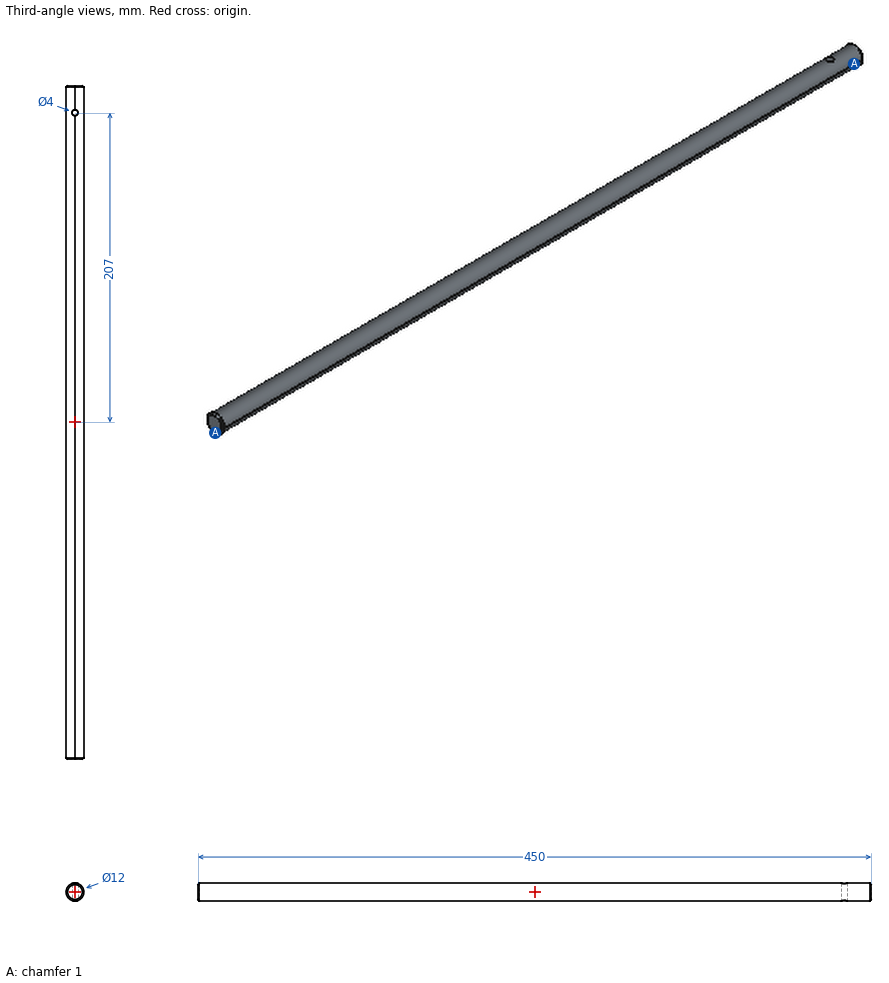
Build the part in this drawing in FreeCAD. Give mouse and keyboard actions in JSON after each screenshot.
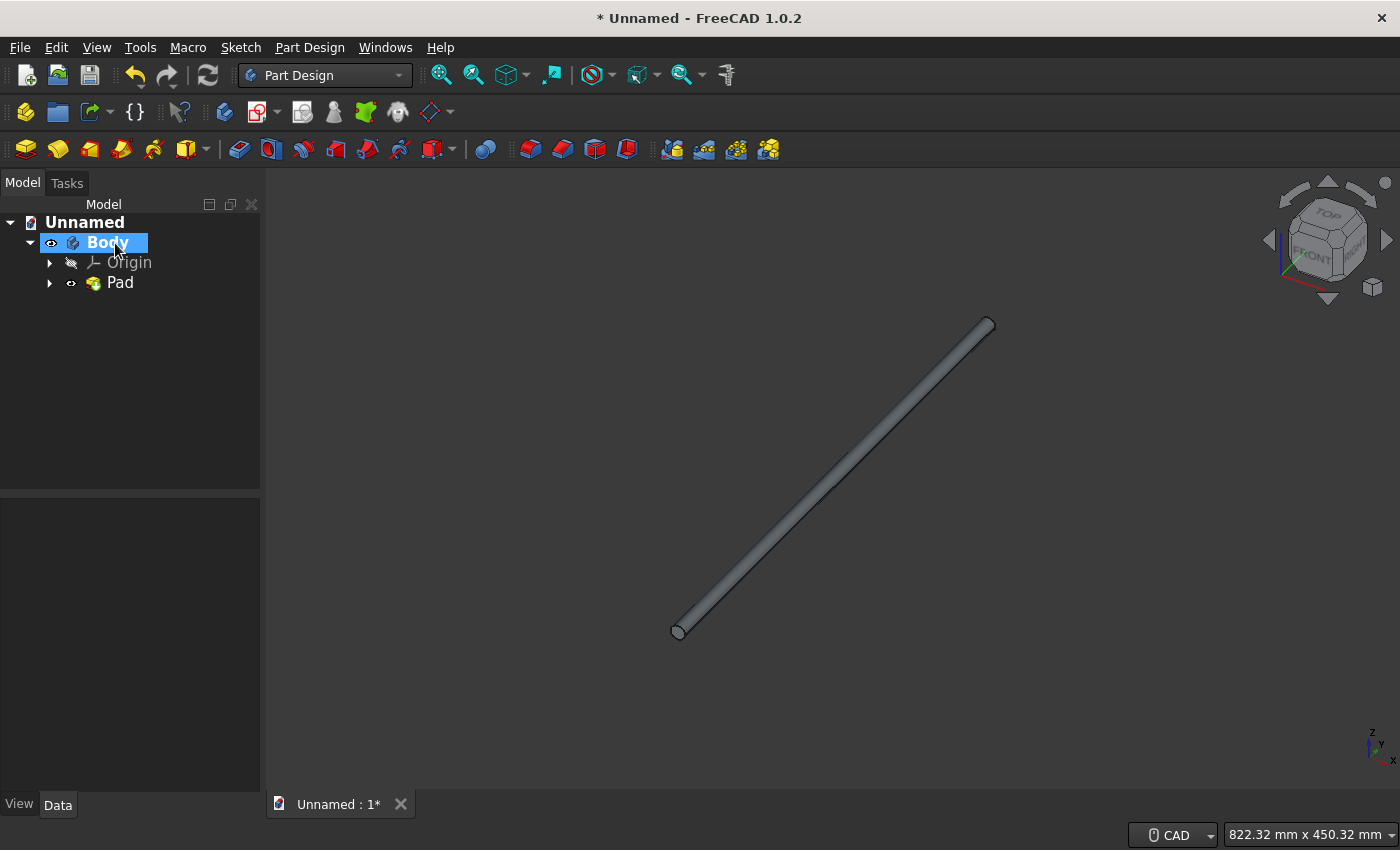
{"action": "left_click", "coordinate": [671, 629]}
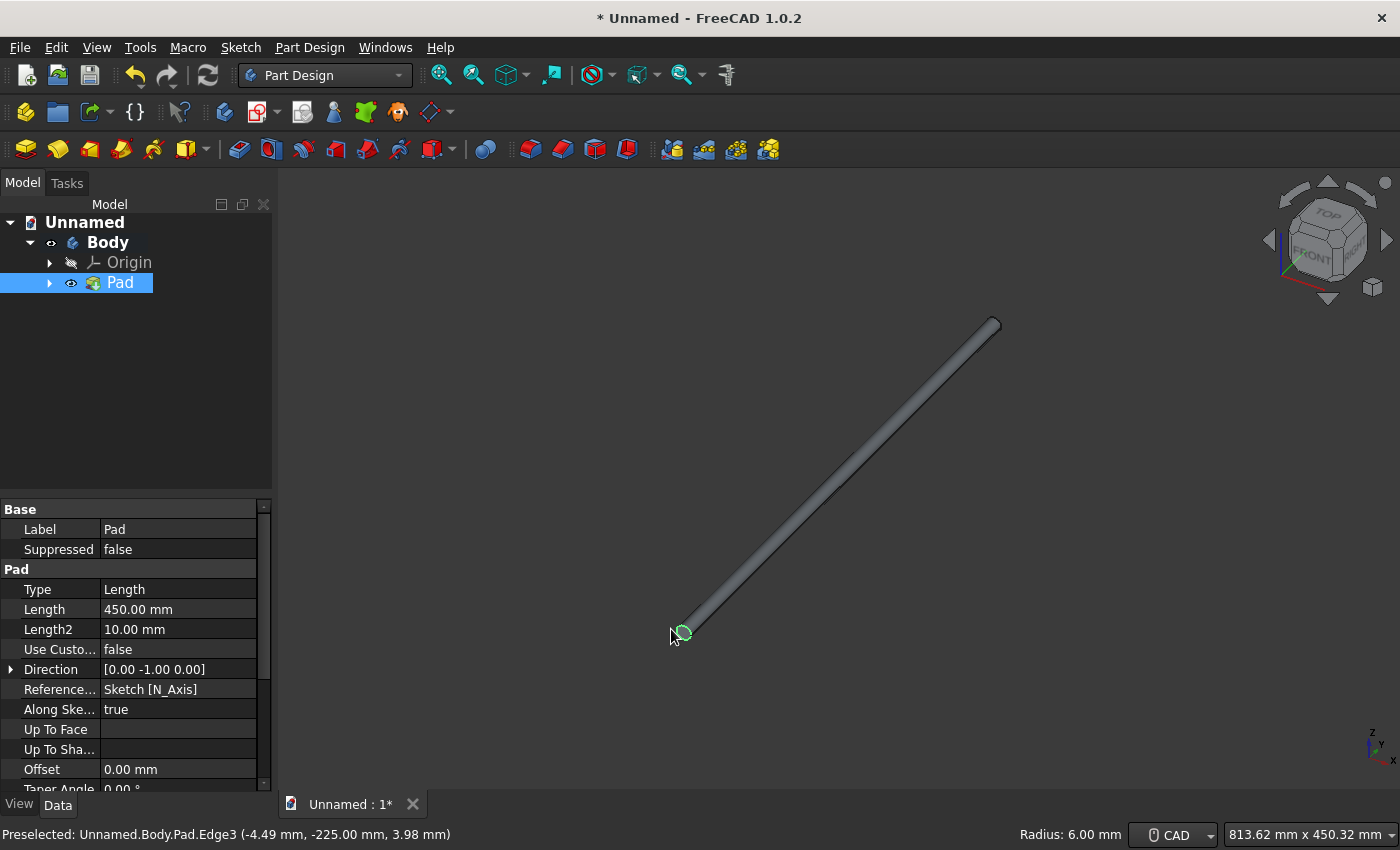
{"action": "left_click", "coordinate": [992, 316], "text": "ctrl"}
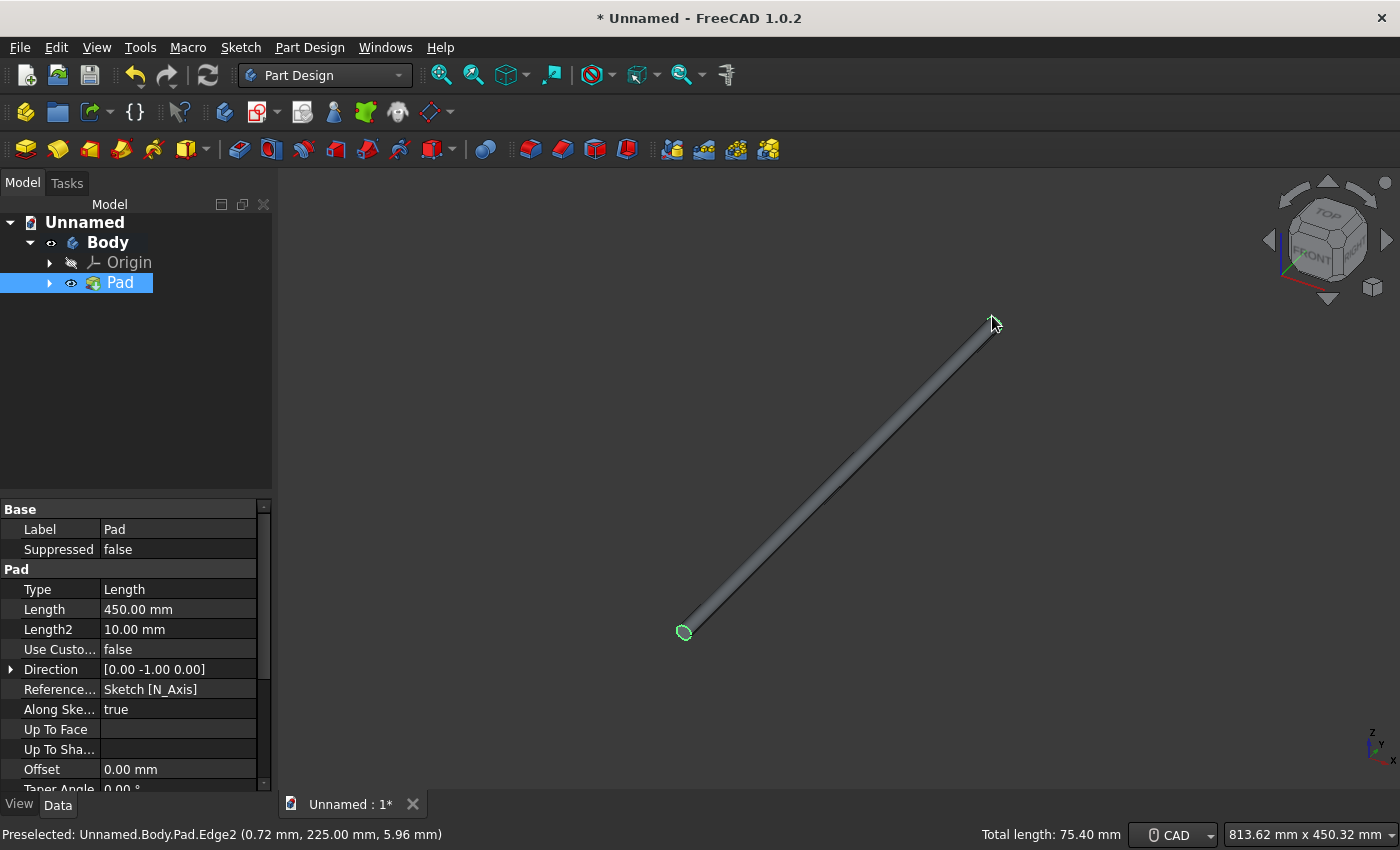
{"action": "left_click", "coordinate": [564, 150]}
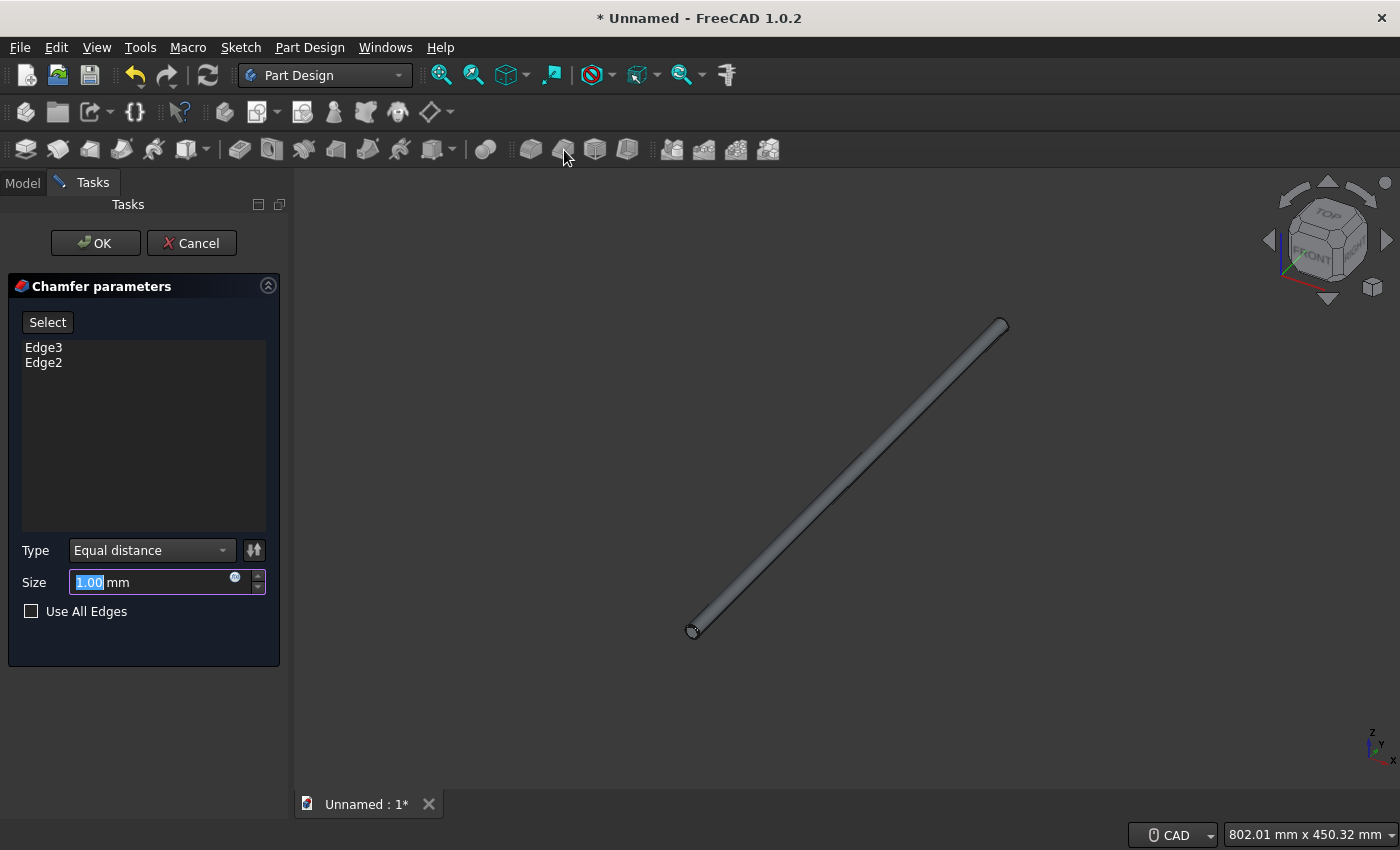
{"action": "type", "text": "1"}
{"action": "key", "text": "Tab"}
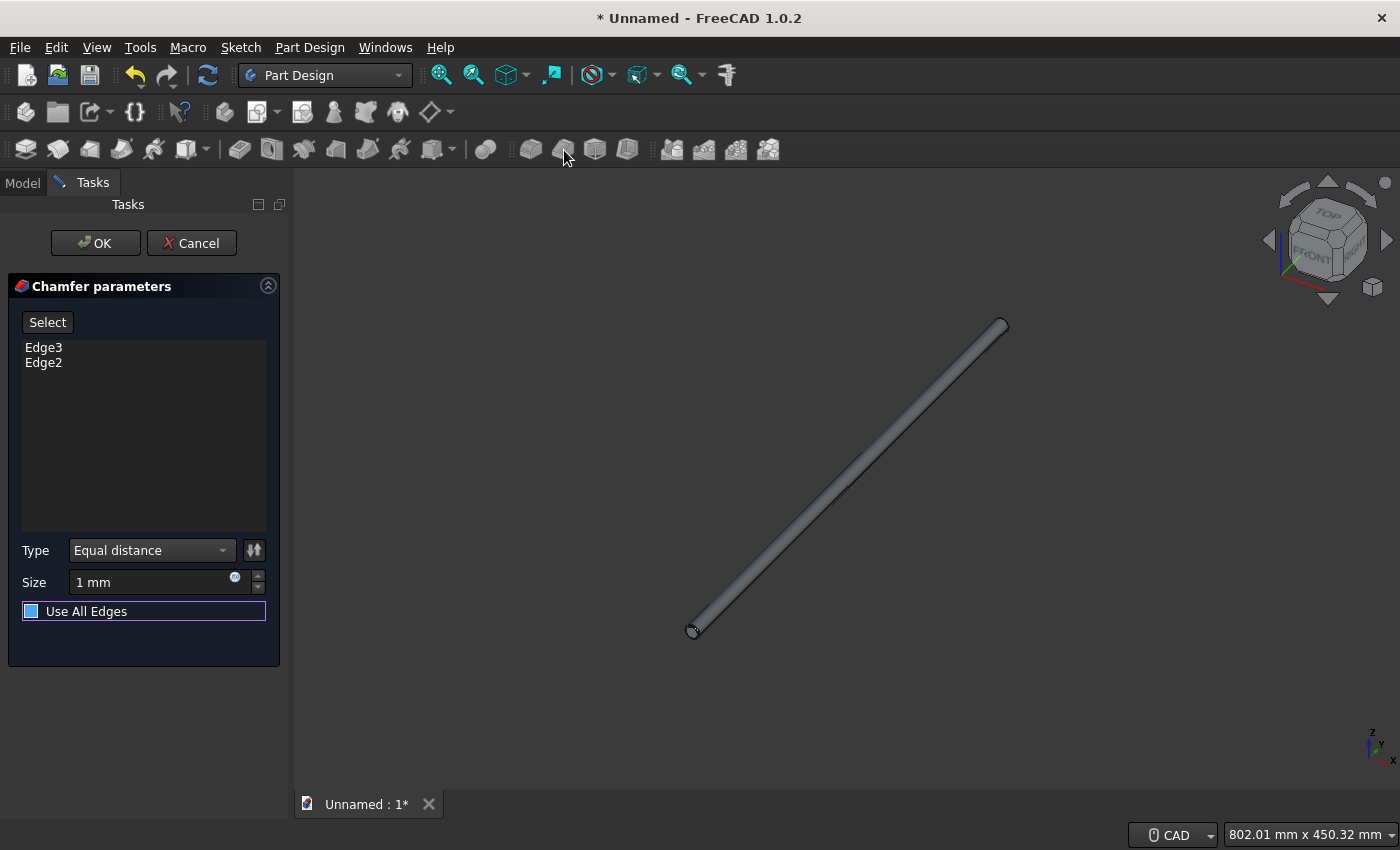
{"action": "left_click", "coordinate": [96, 243]}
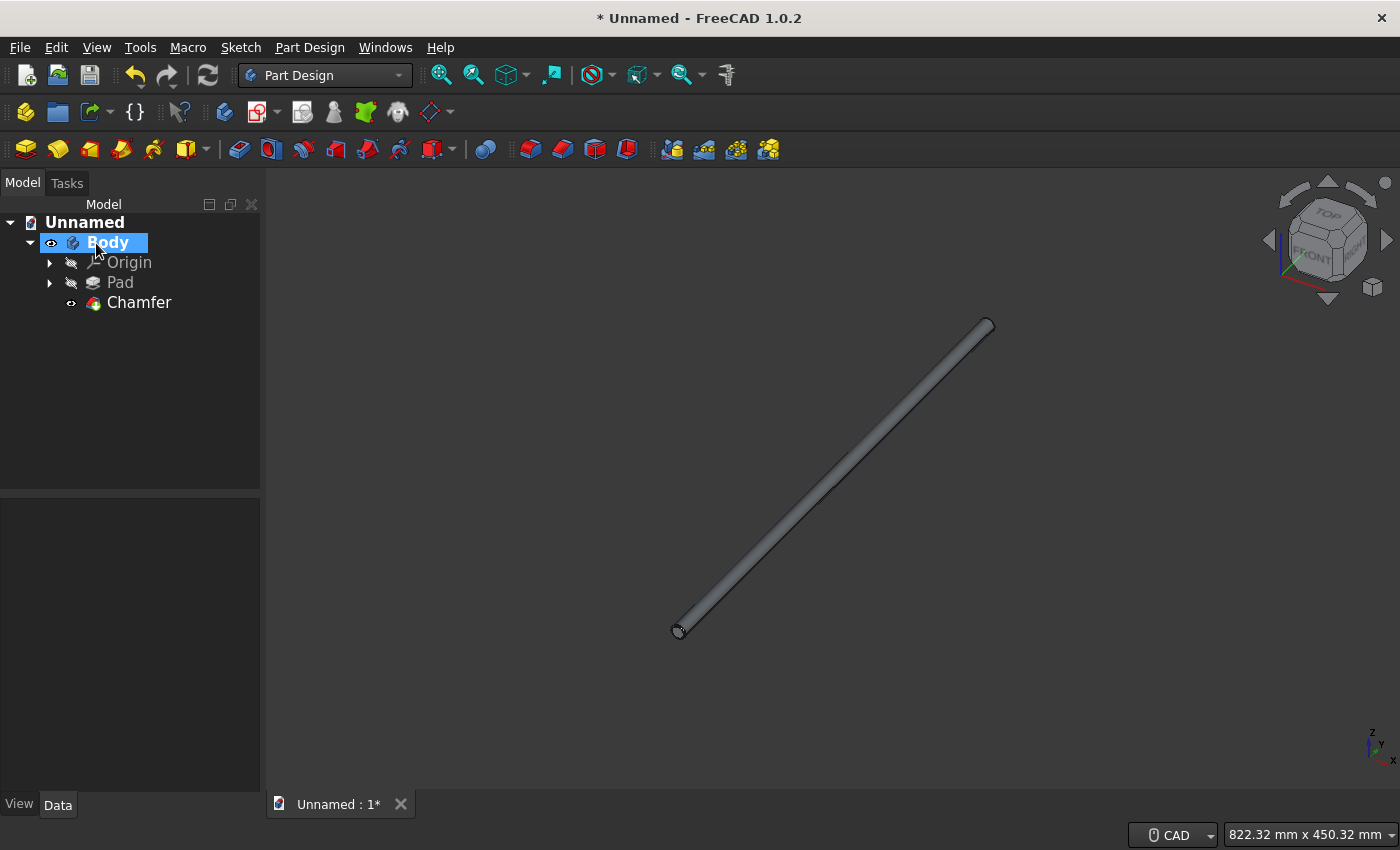
{"action": "left_click", "coordinate": [258, 112]}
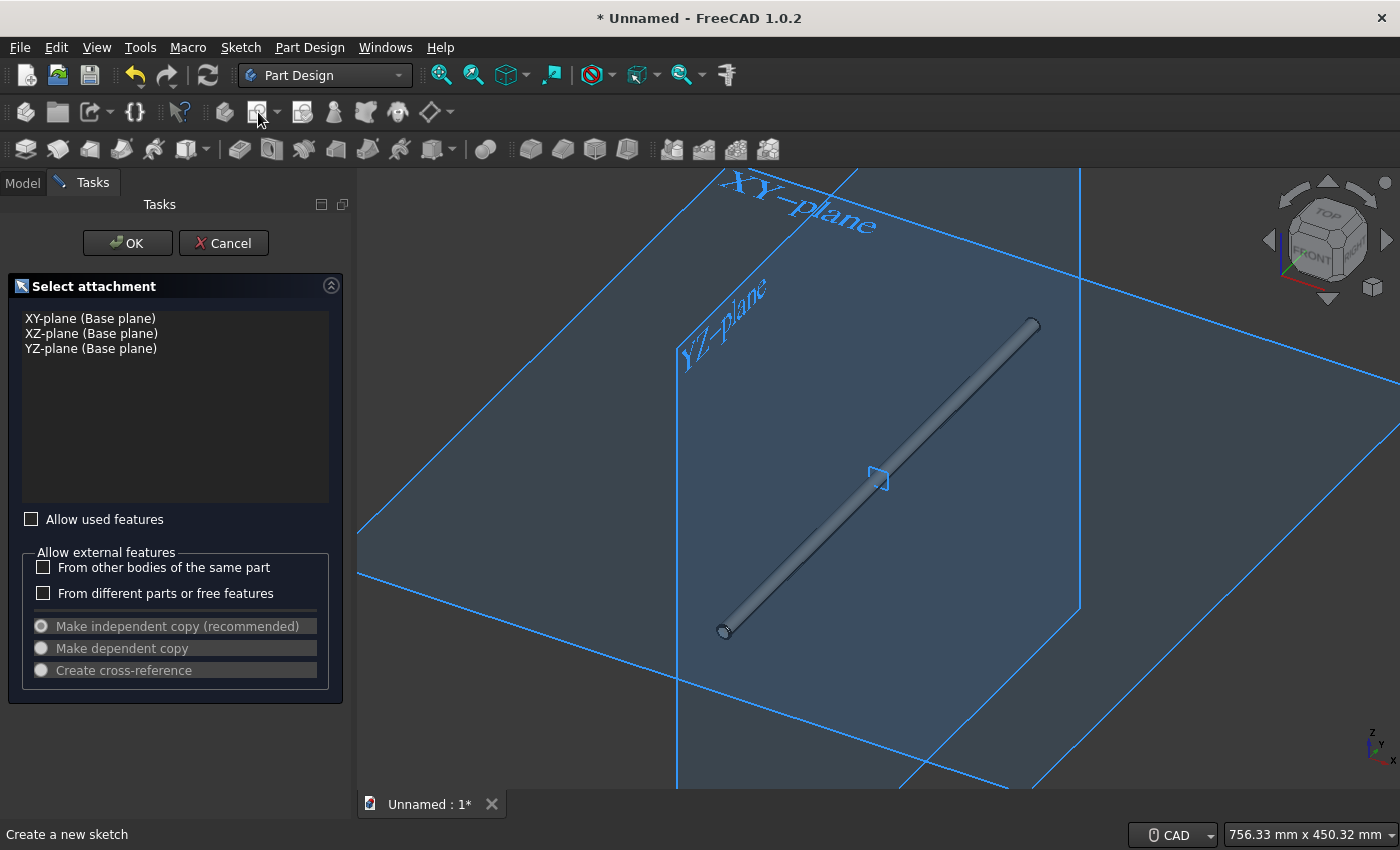
{"action": "left_click", "coordinate": [82, 318]}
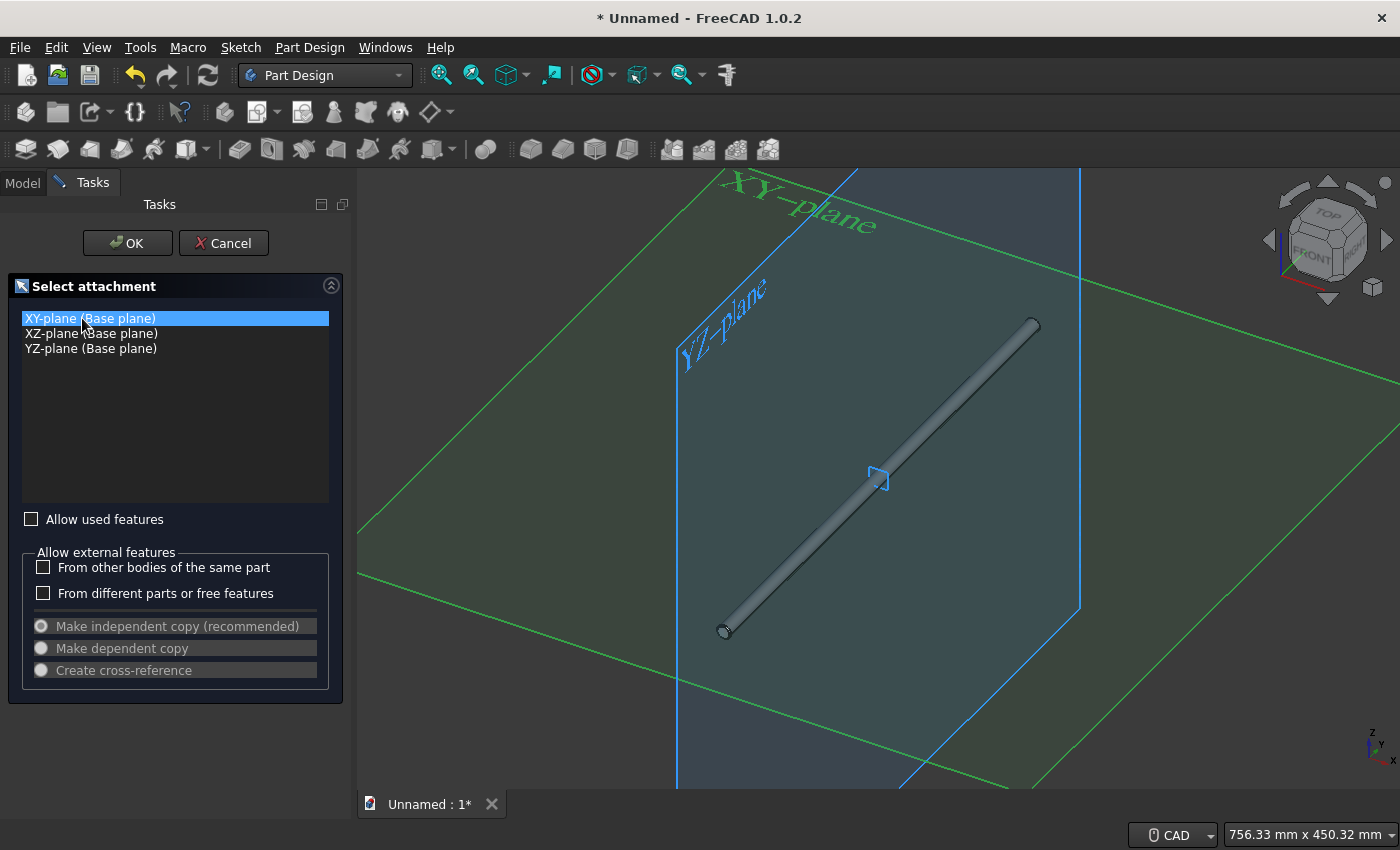
{"action": "left_click", "coordinate": [128, 243]}